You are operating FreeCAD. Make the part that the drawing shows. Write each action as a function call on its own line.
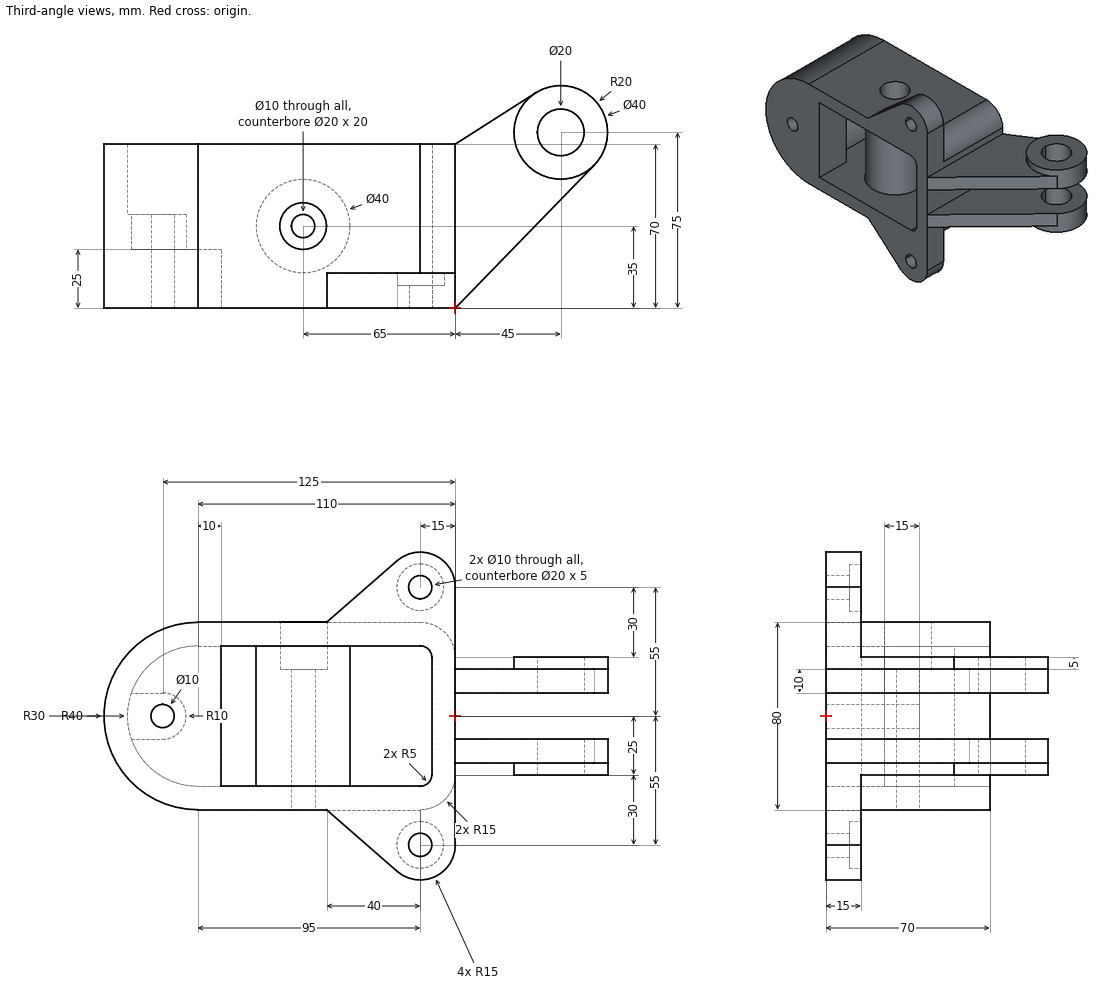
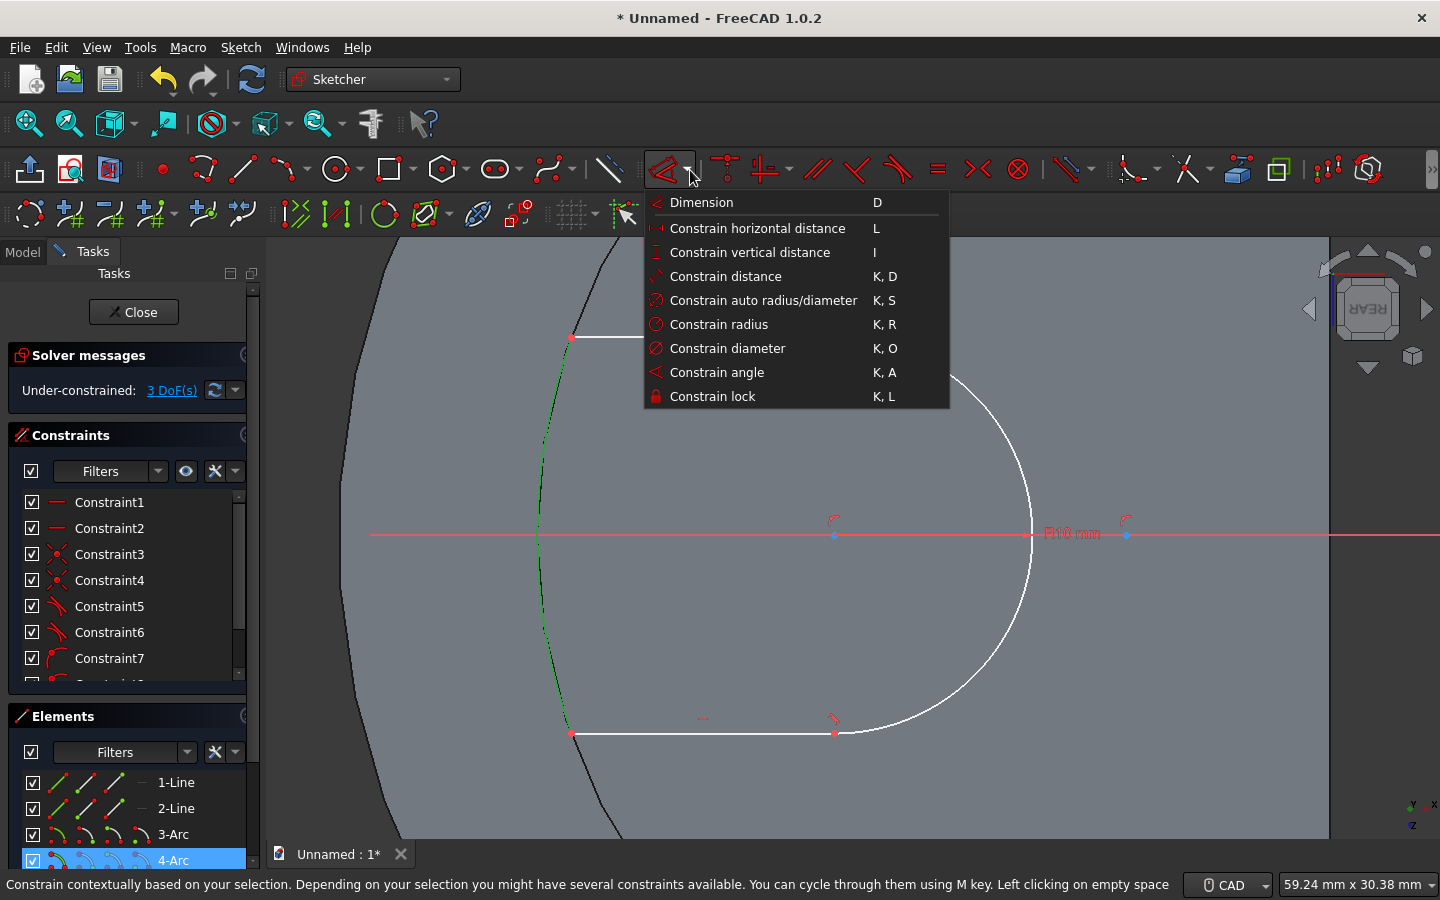
click(797, 324)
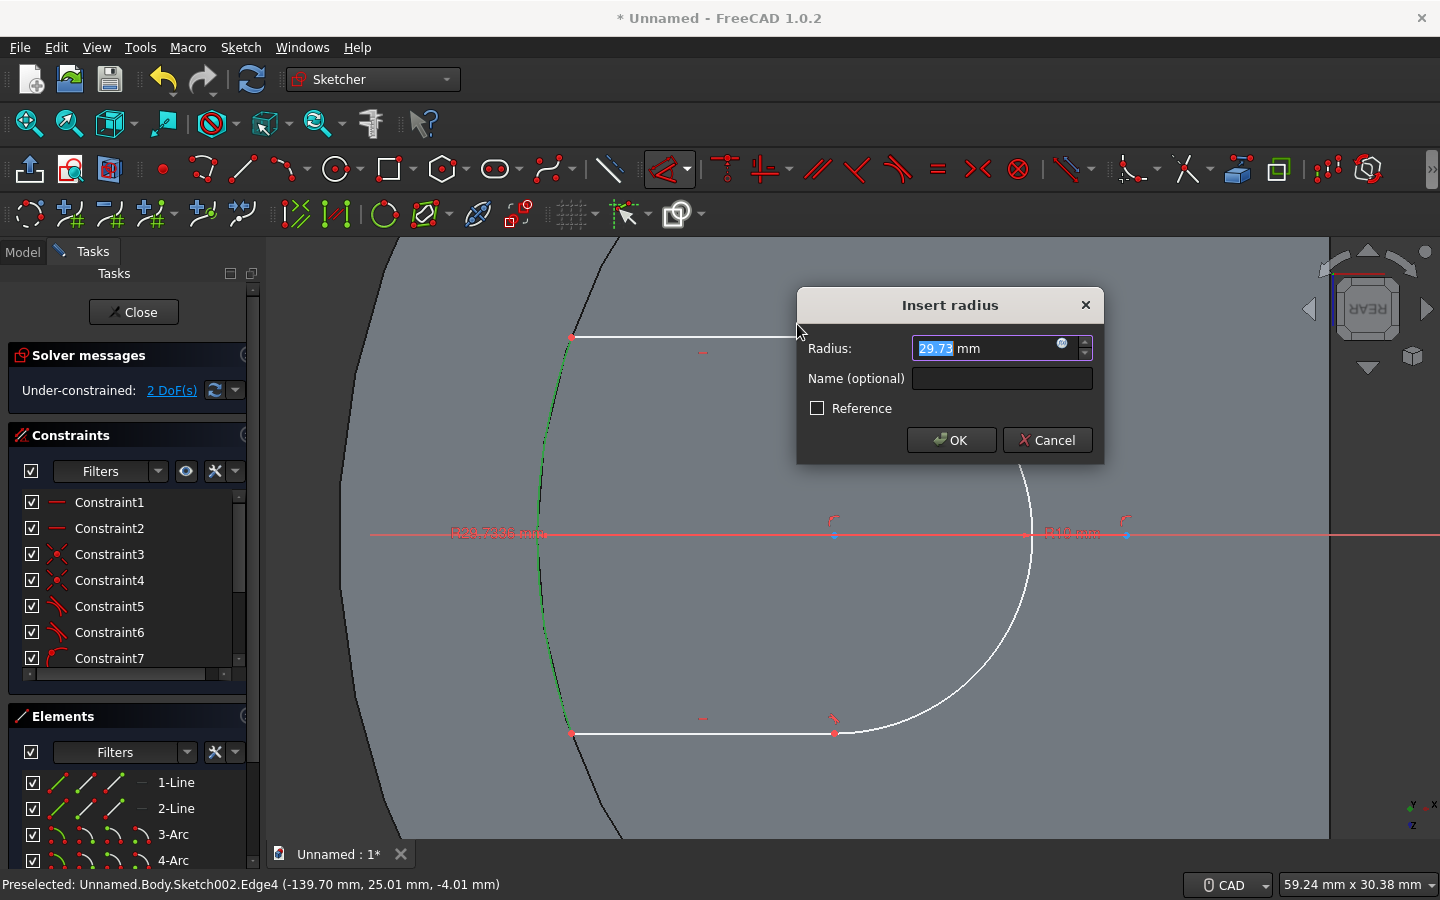
text(30)
key(Return)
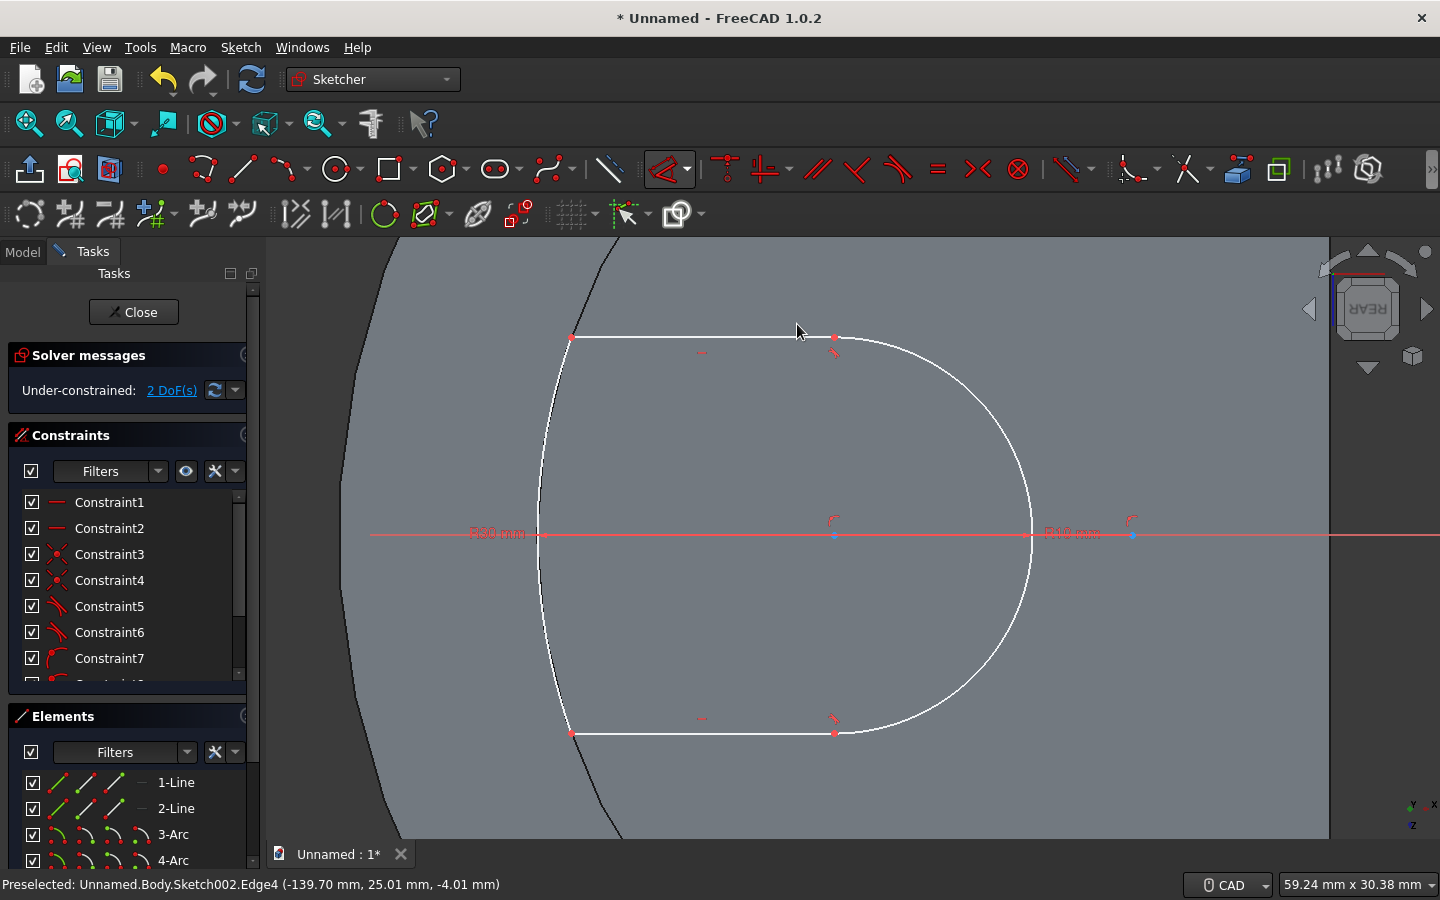
click(834, 734)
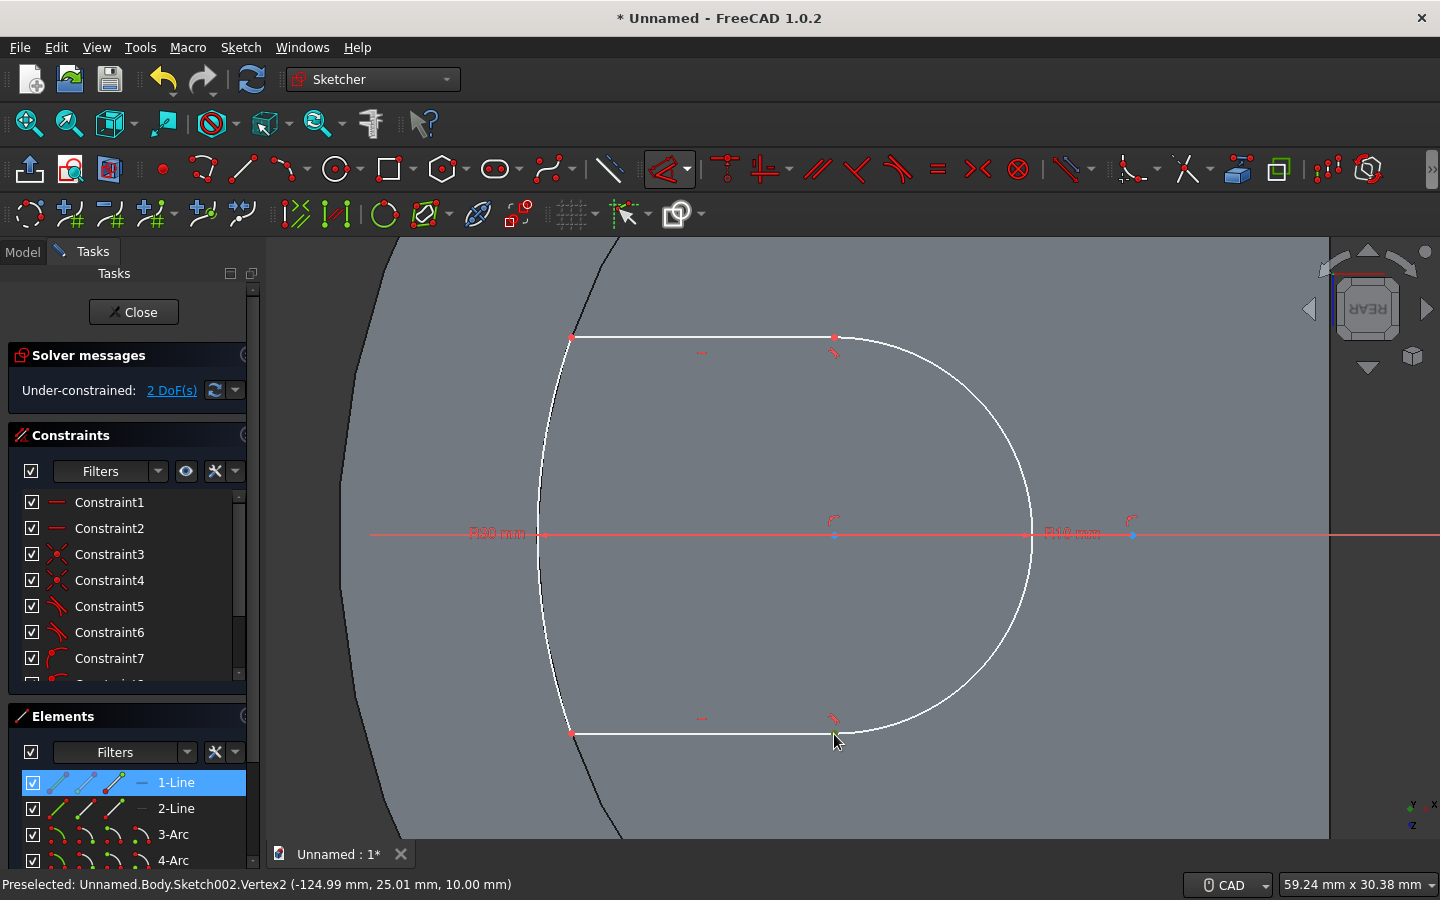
key(l)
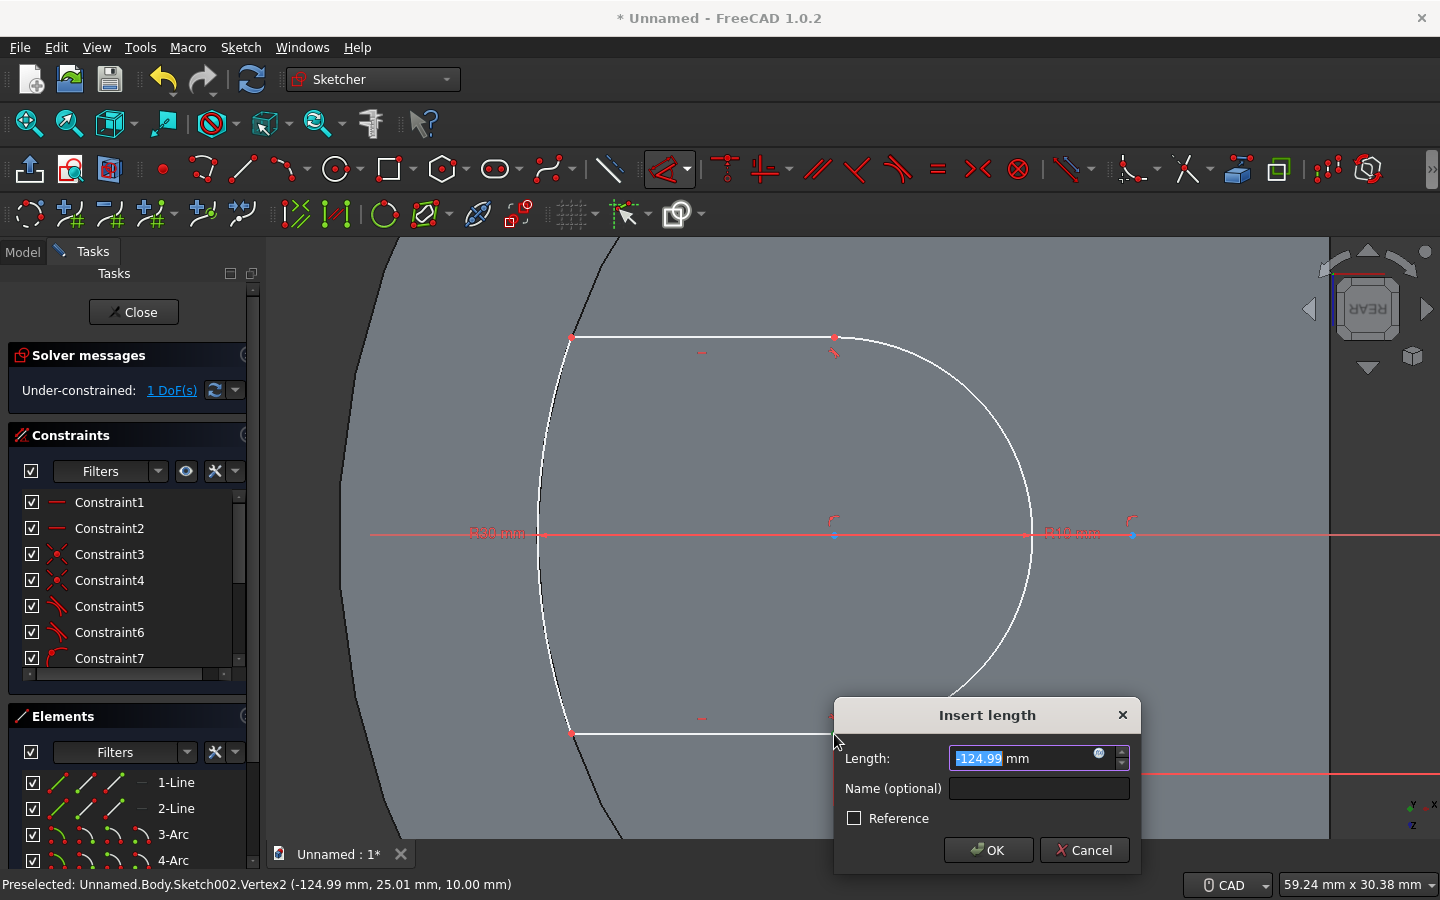
text(-125)
key(Return)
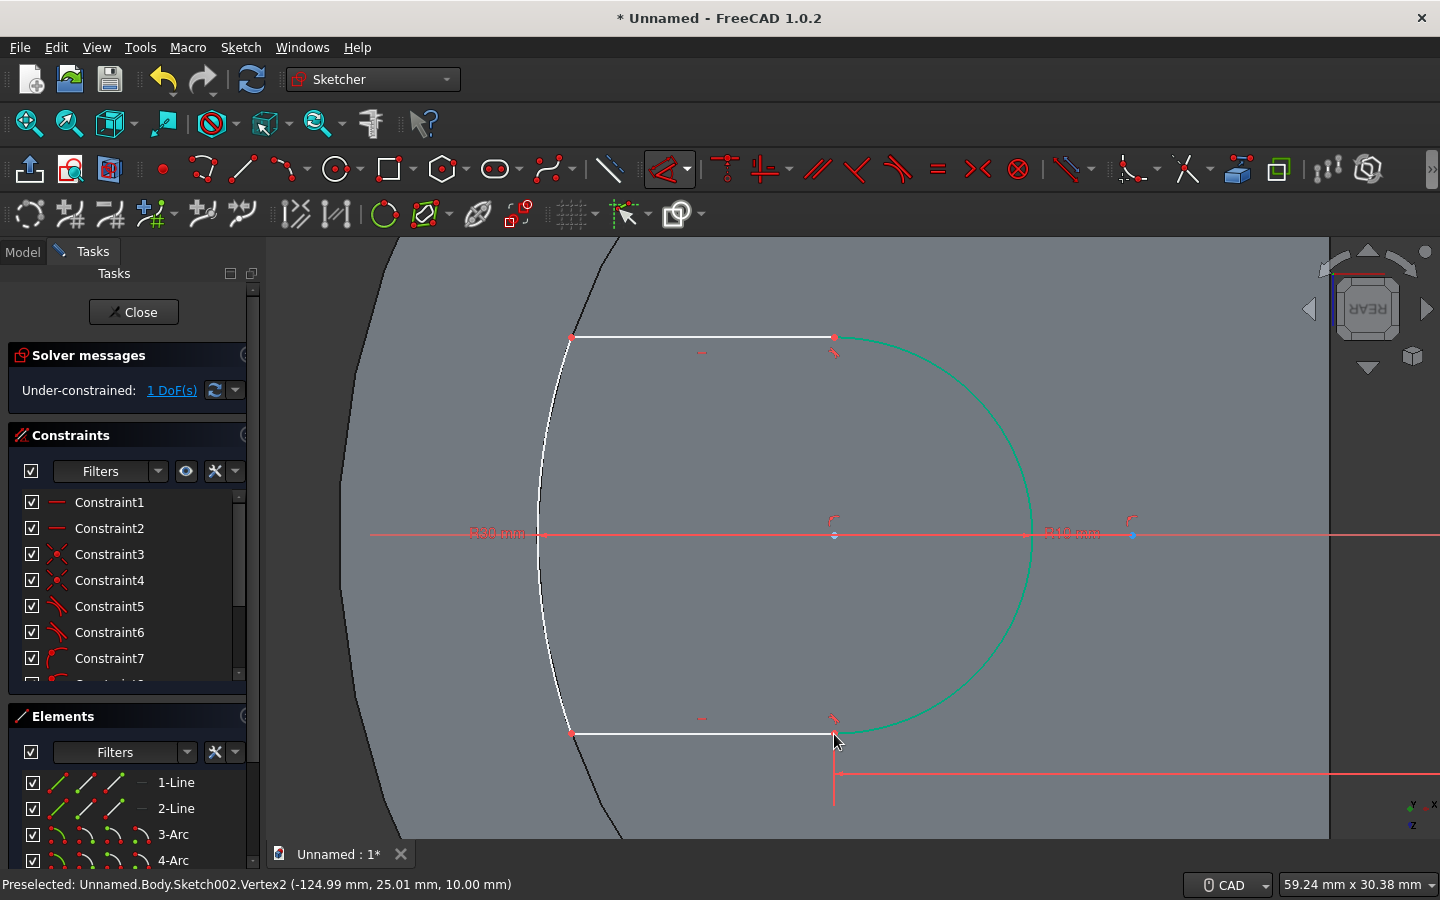
click(1132, 535)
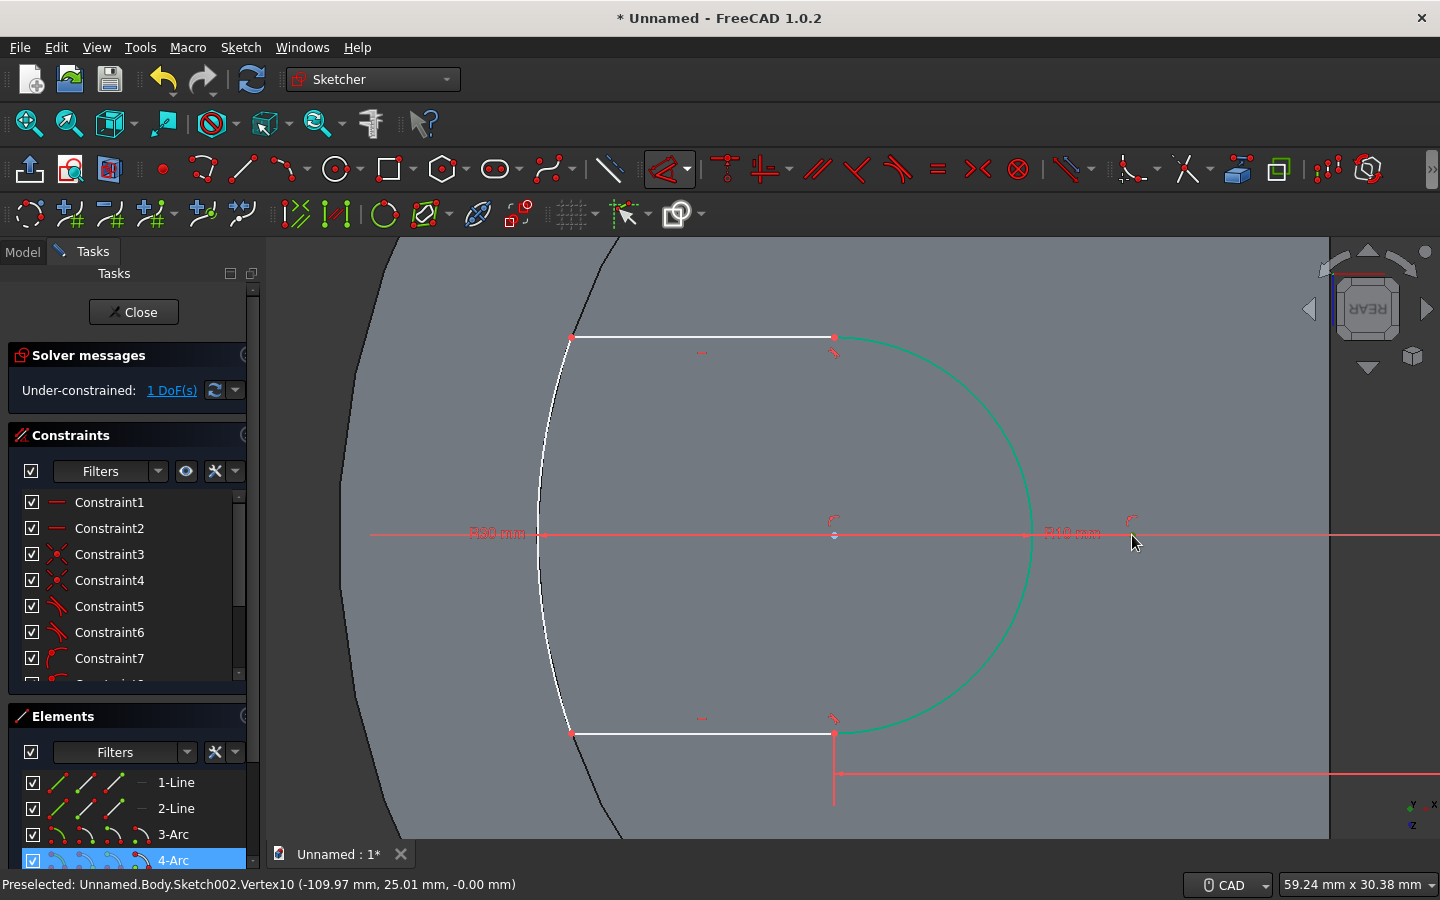
key(l)